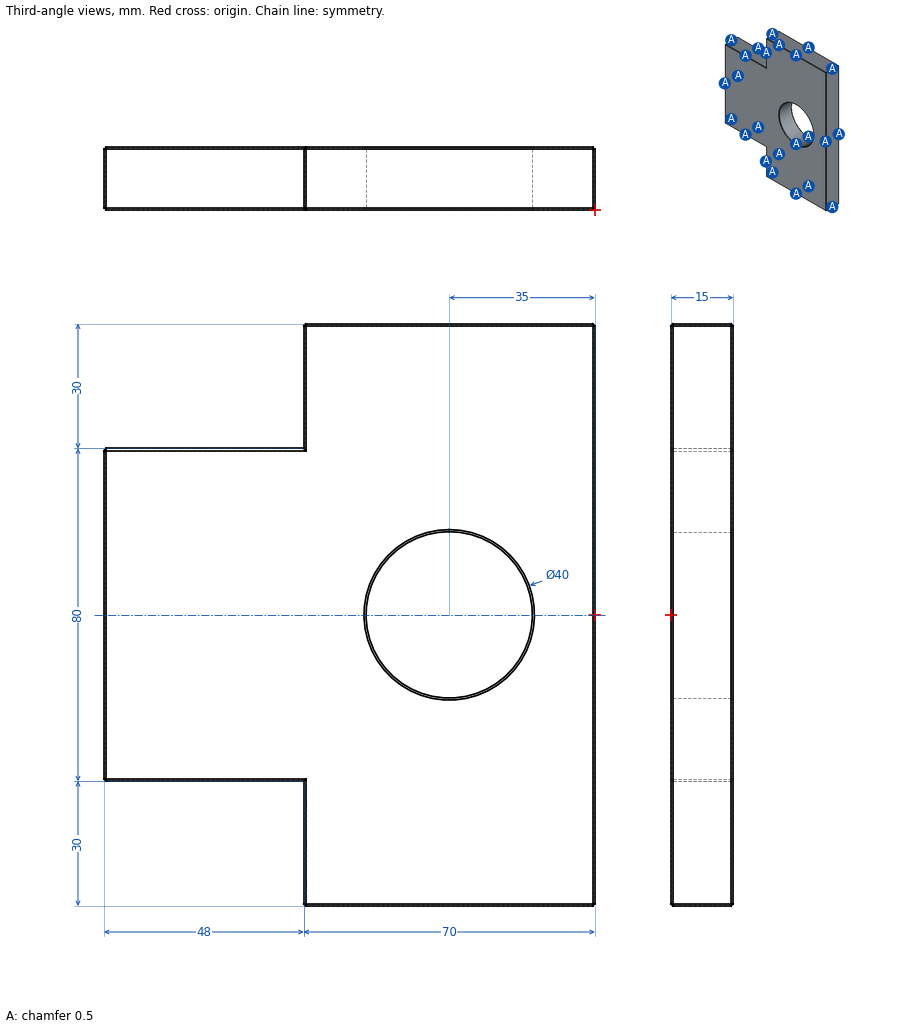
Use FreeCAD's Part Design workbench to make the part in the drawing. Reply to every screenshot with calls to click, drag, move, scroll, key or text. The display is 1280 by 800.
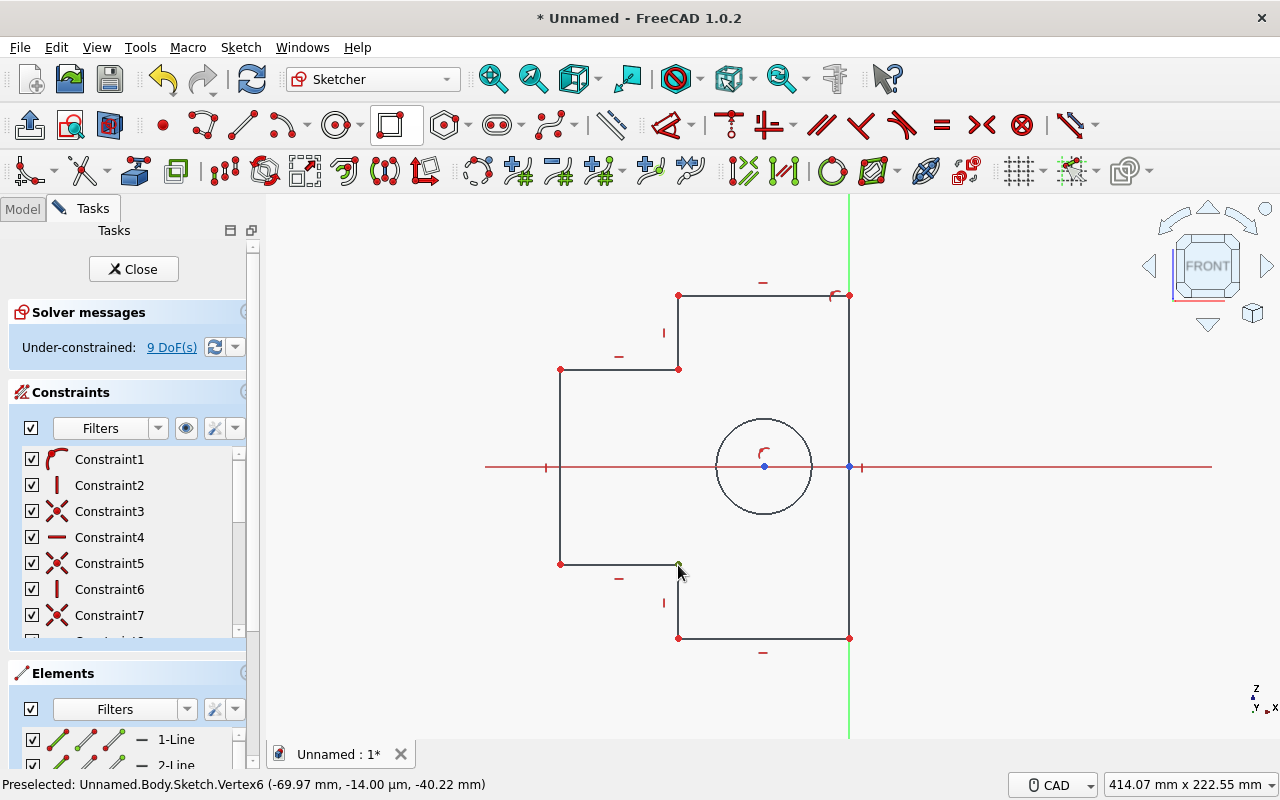
click(678, 370)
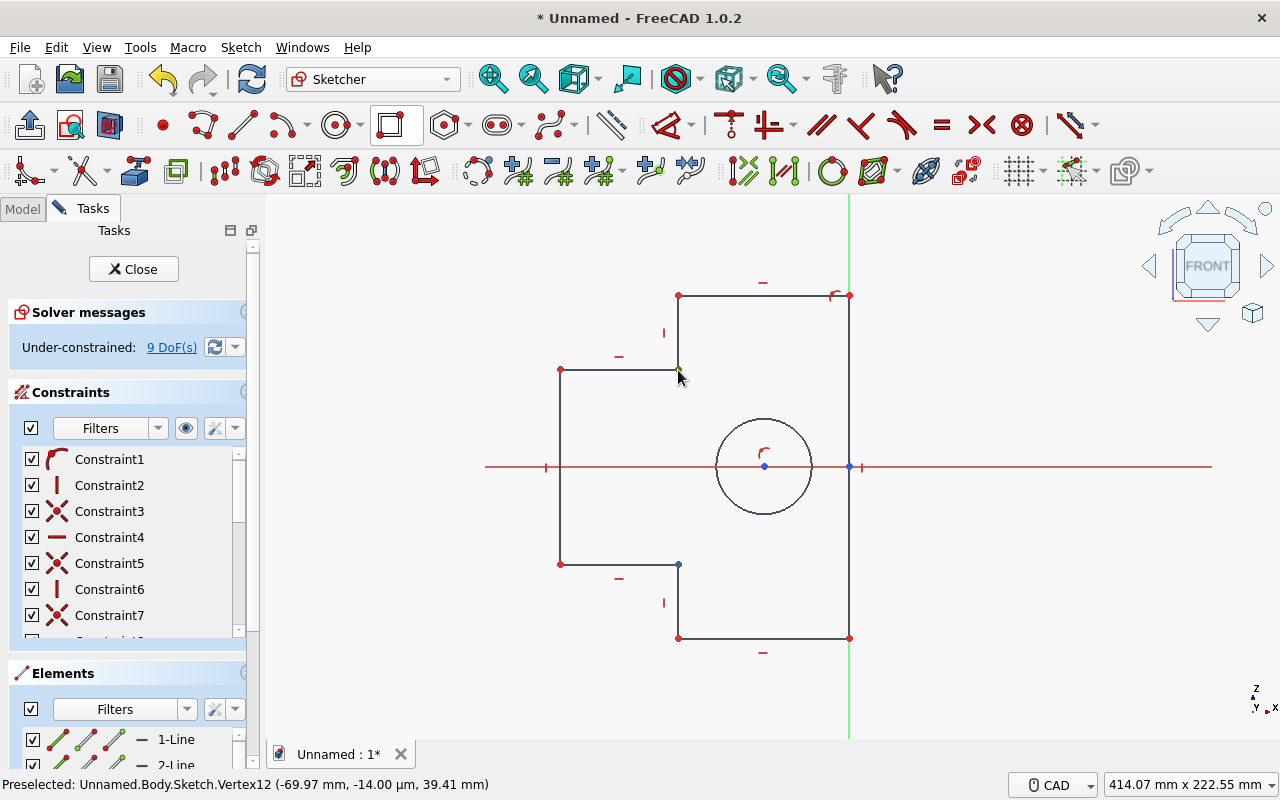
click(529, 466)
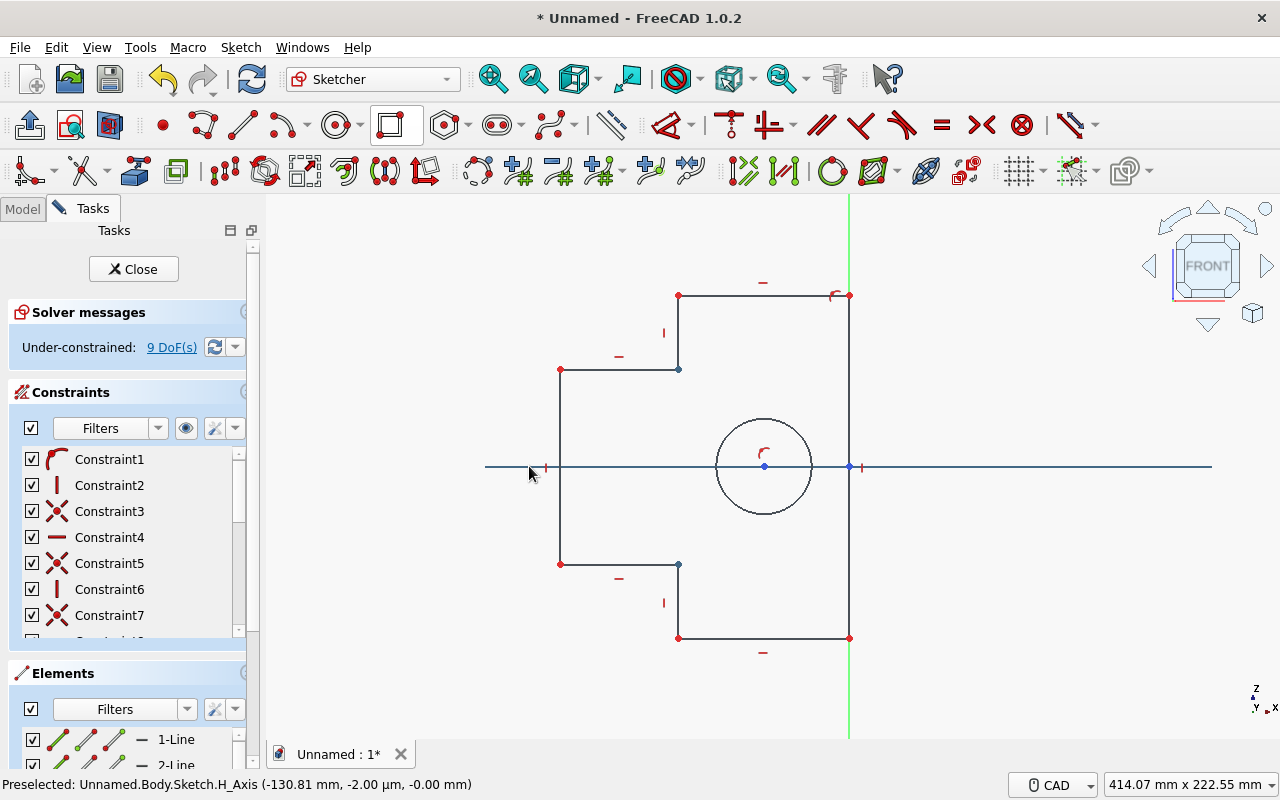
click(982, 126)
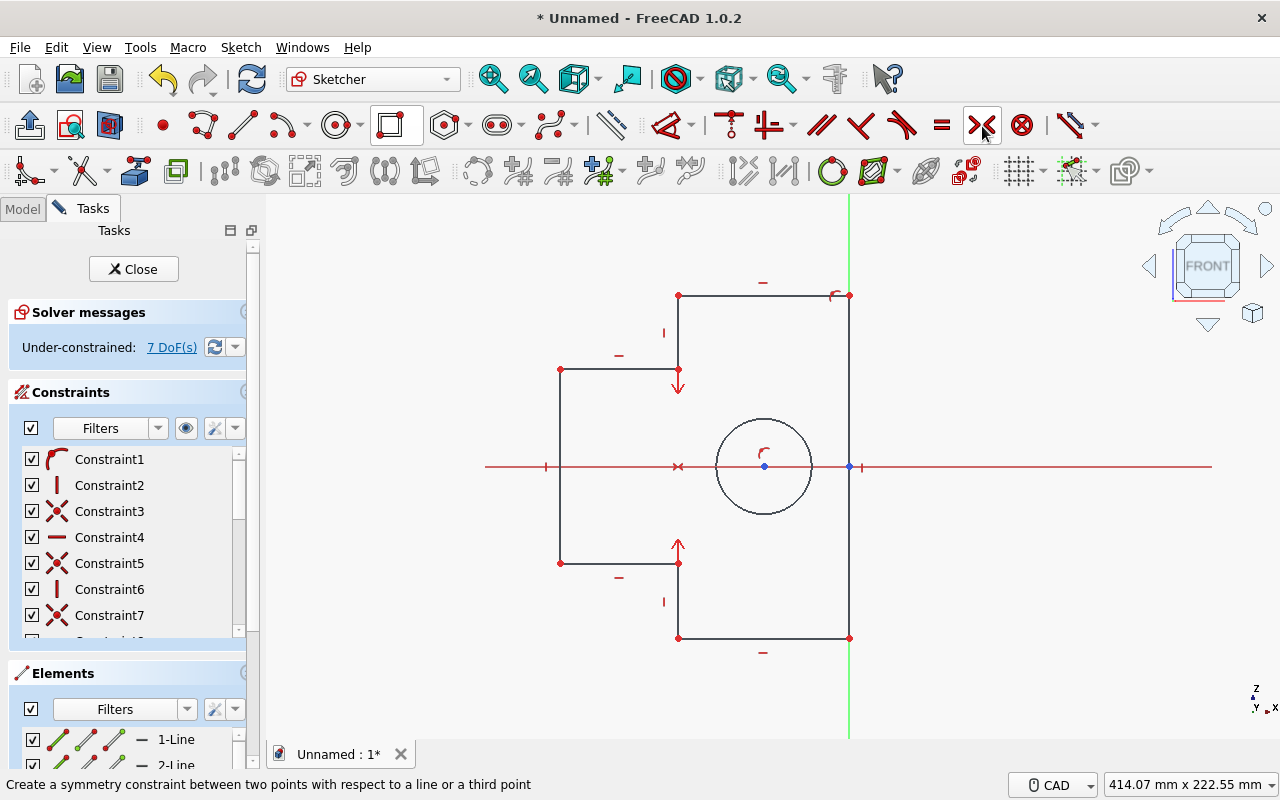
key(d)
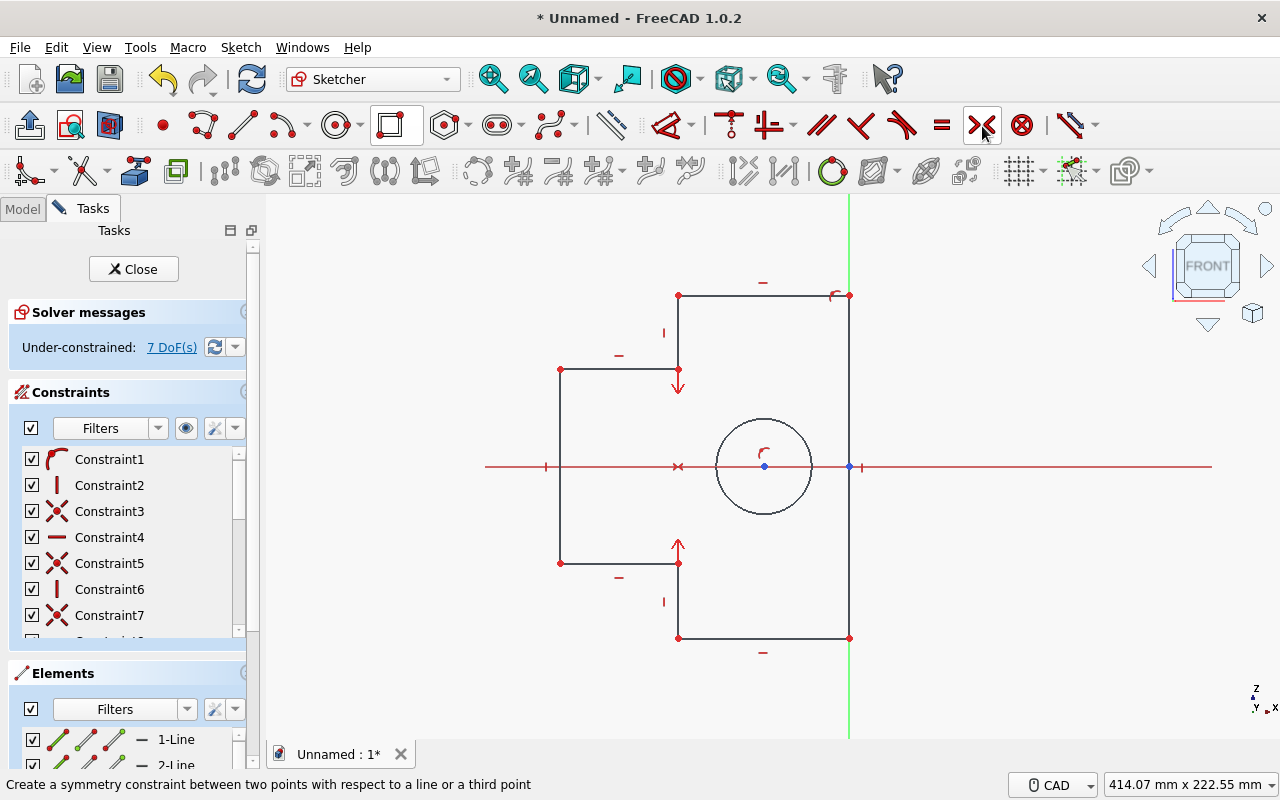
click(798, 433)
click(821, 411)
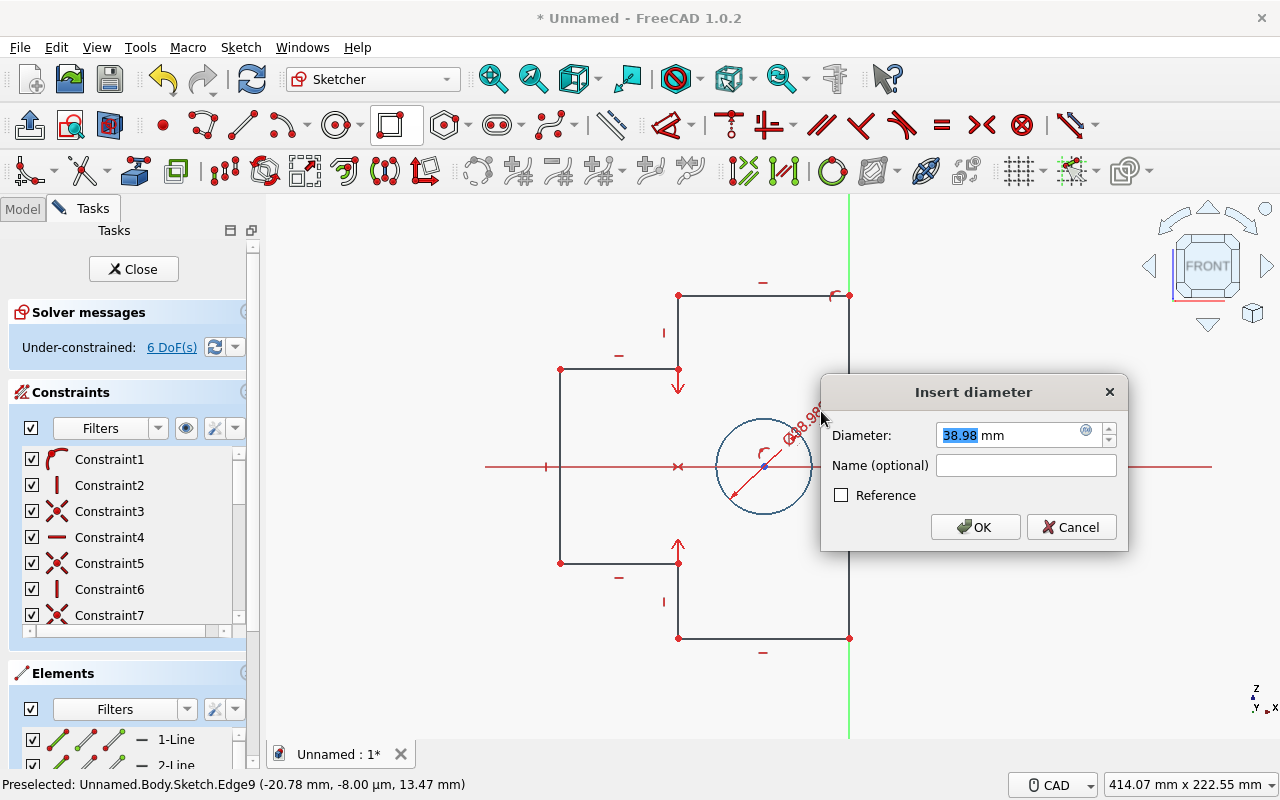
text(40)
key(Return)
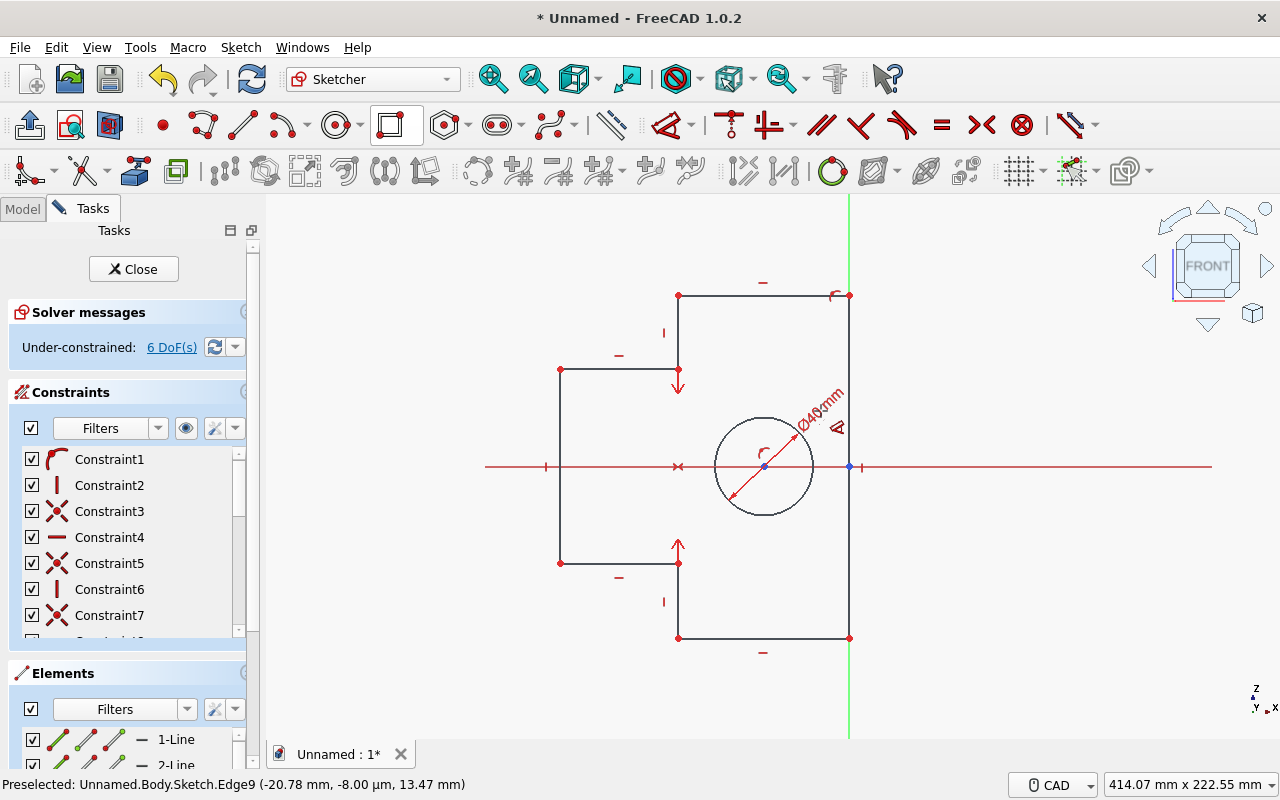
click(798, 639)
click(764, 673)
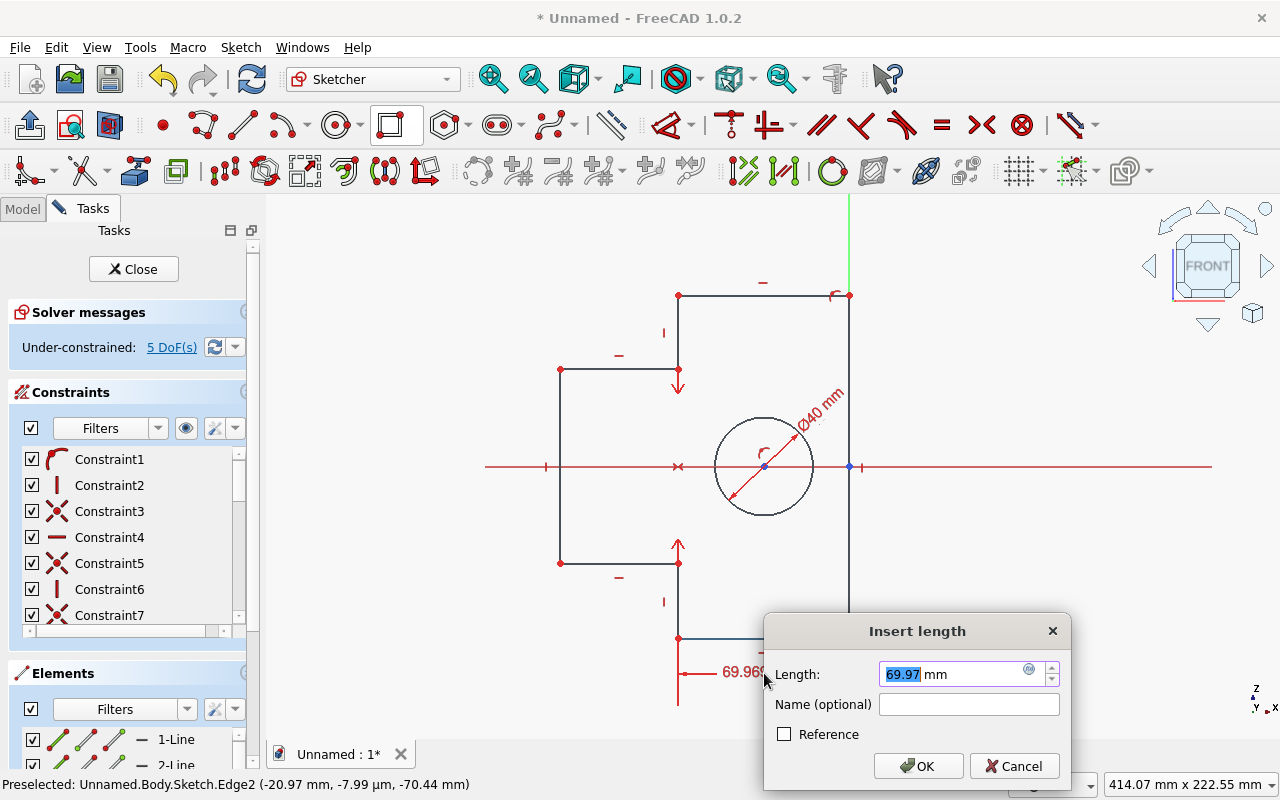
text(70)
key(Return)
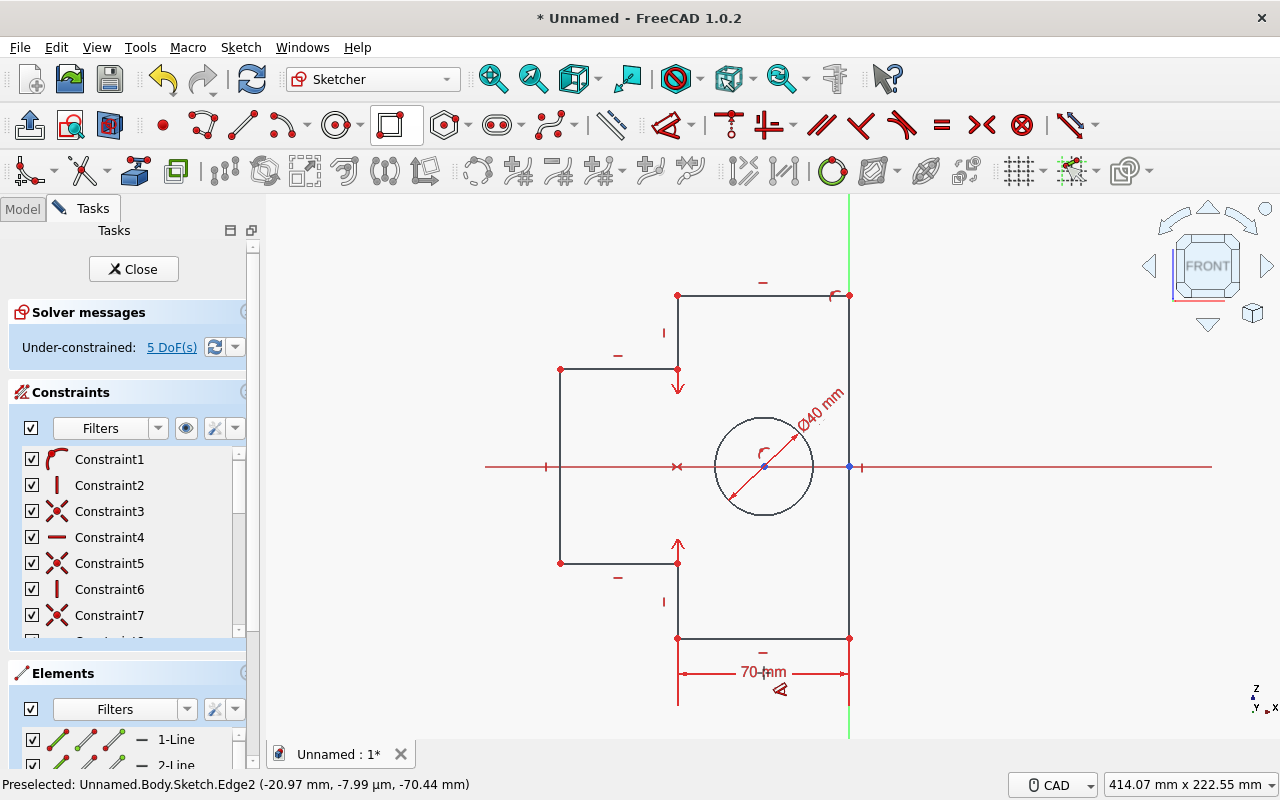
click(678, 616)
click(644, 601)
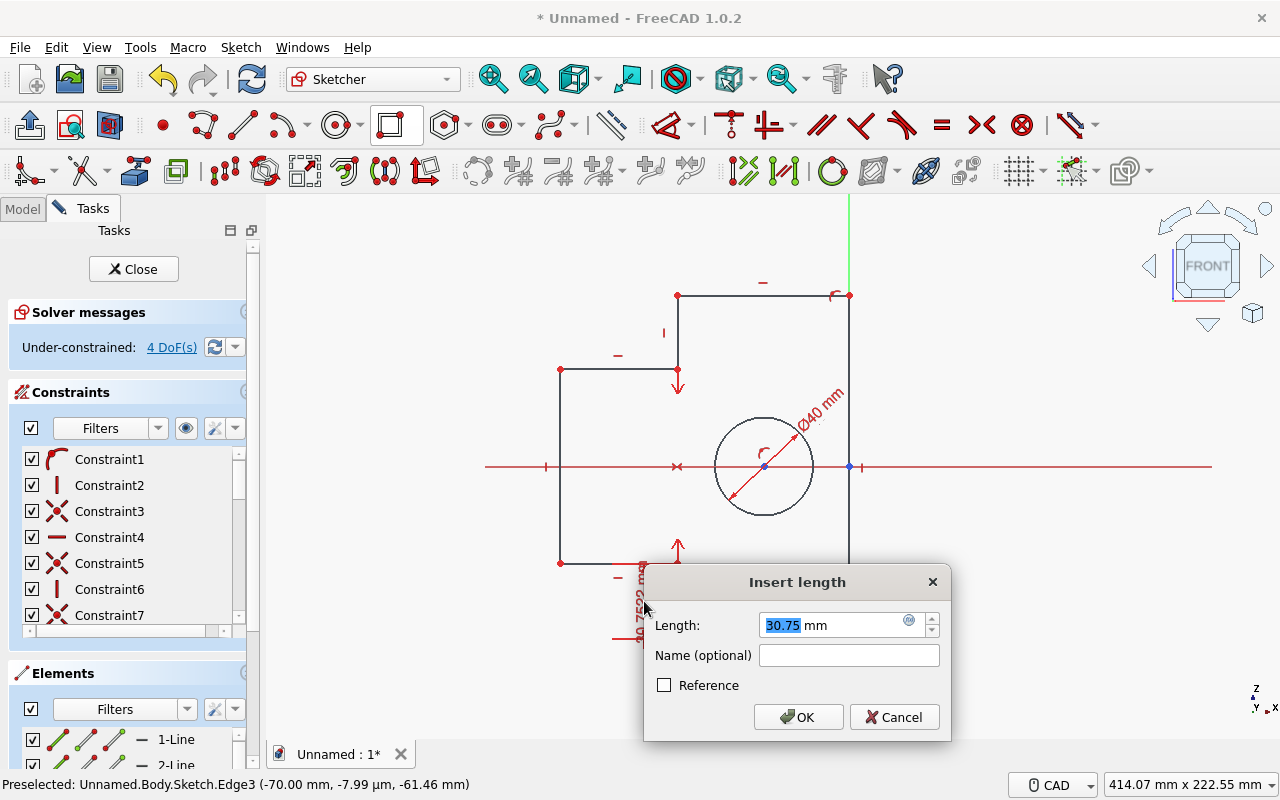
text(30)
key(Return)